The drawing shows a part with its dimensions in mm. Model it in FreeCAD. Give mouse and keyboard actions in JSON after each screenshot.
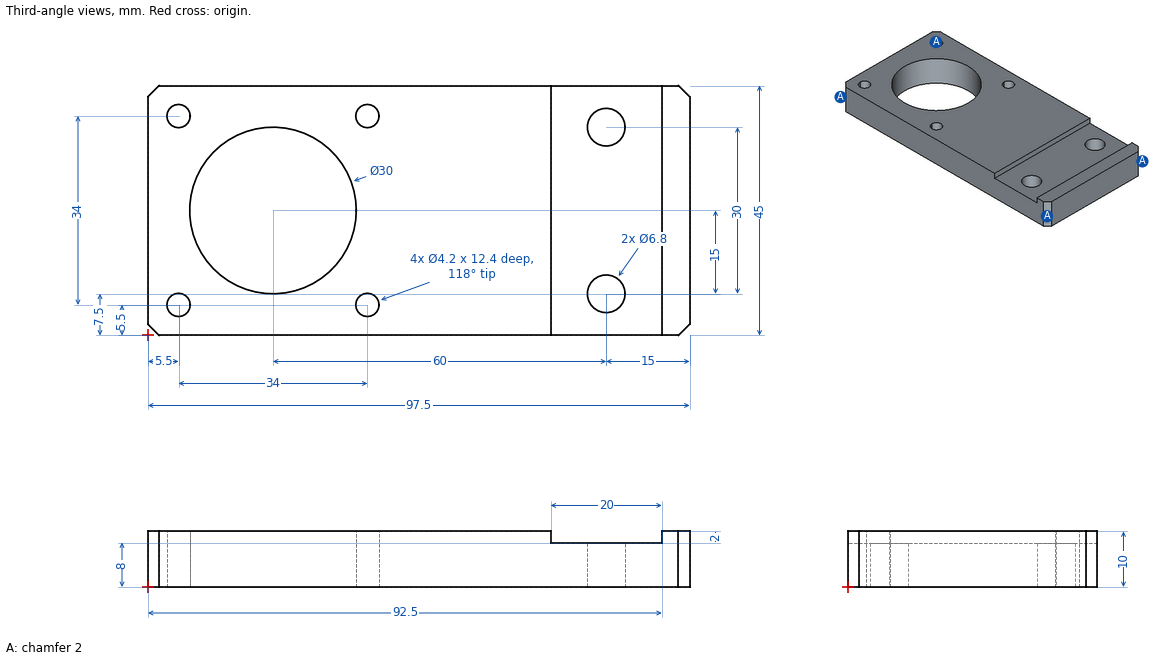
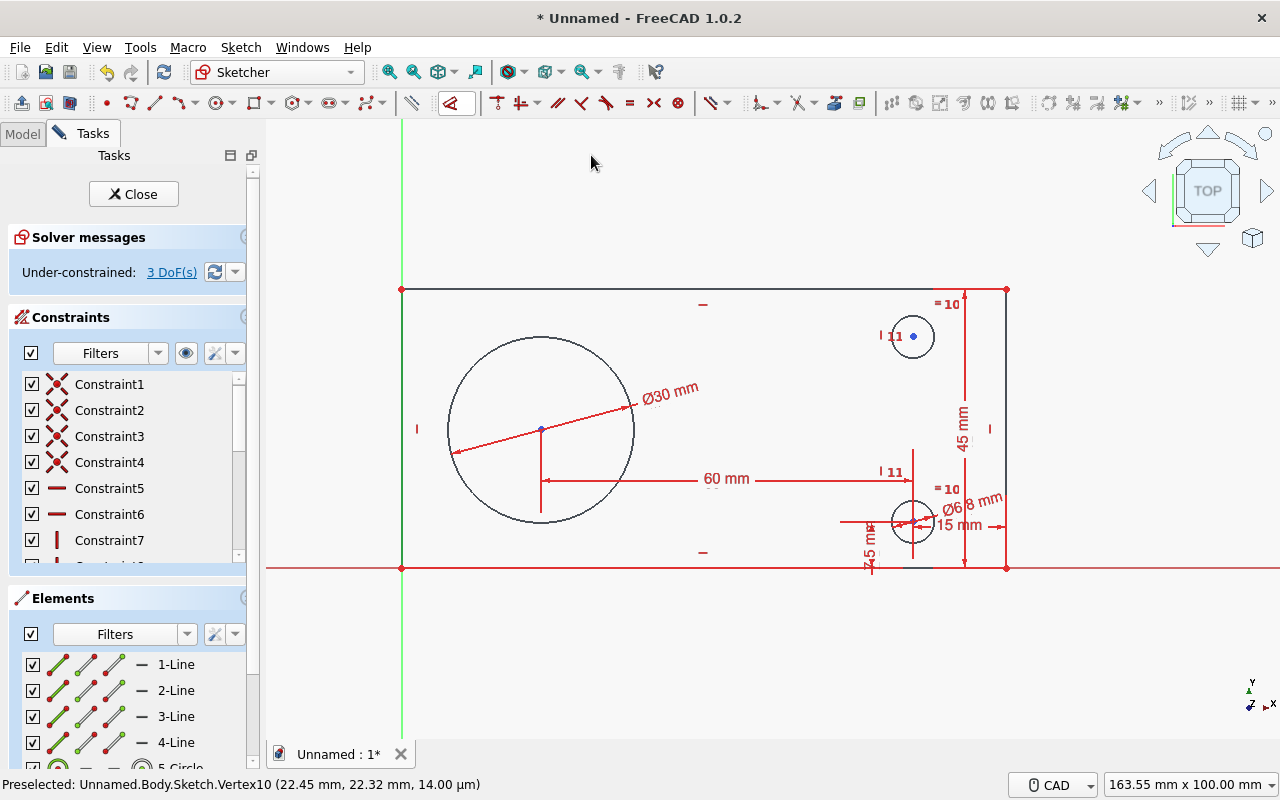
{"action": "left_click", "coordinate": [913, 522]}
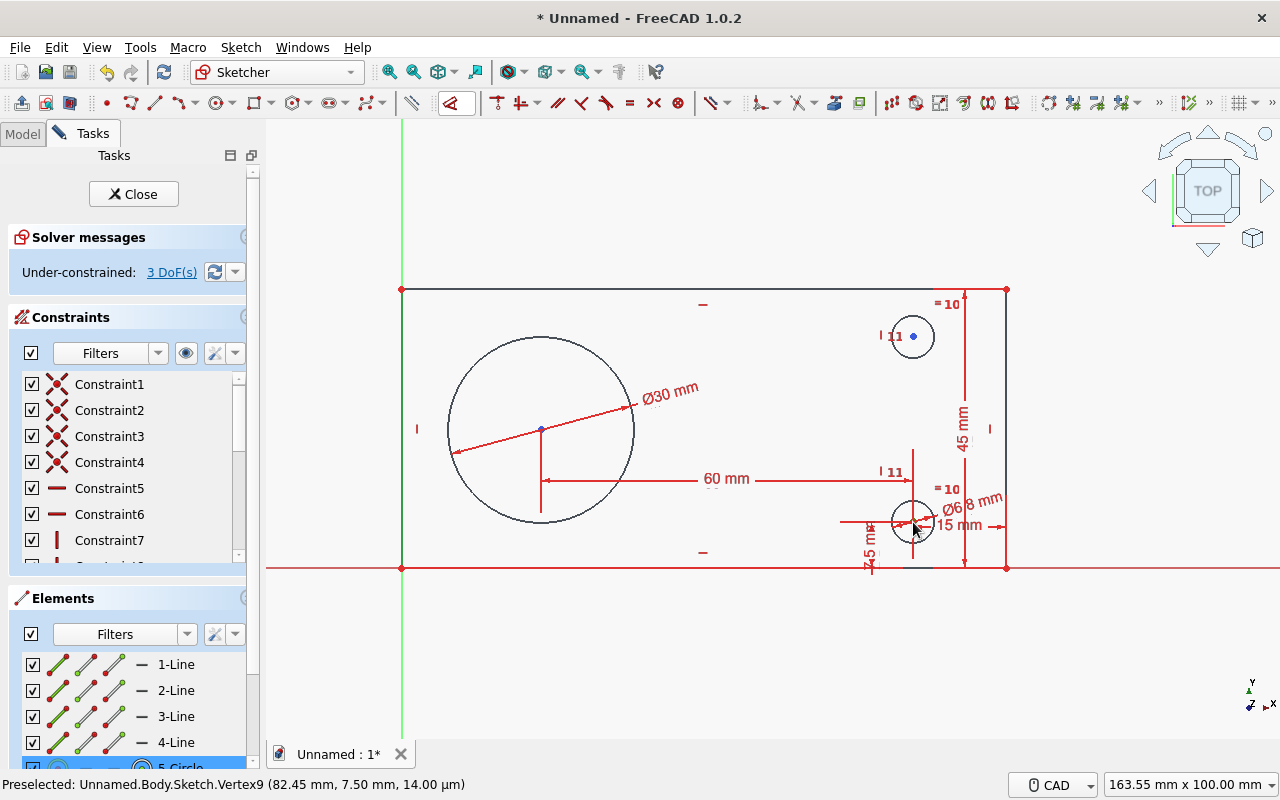
{"action": "left_click", "coordinate": [541, 430]}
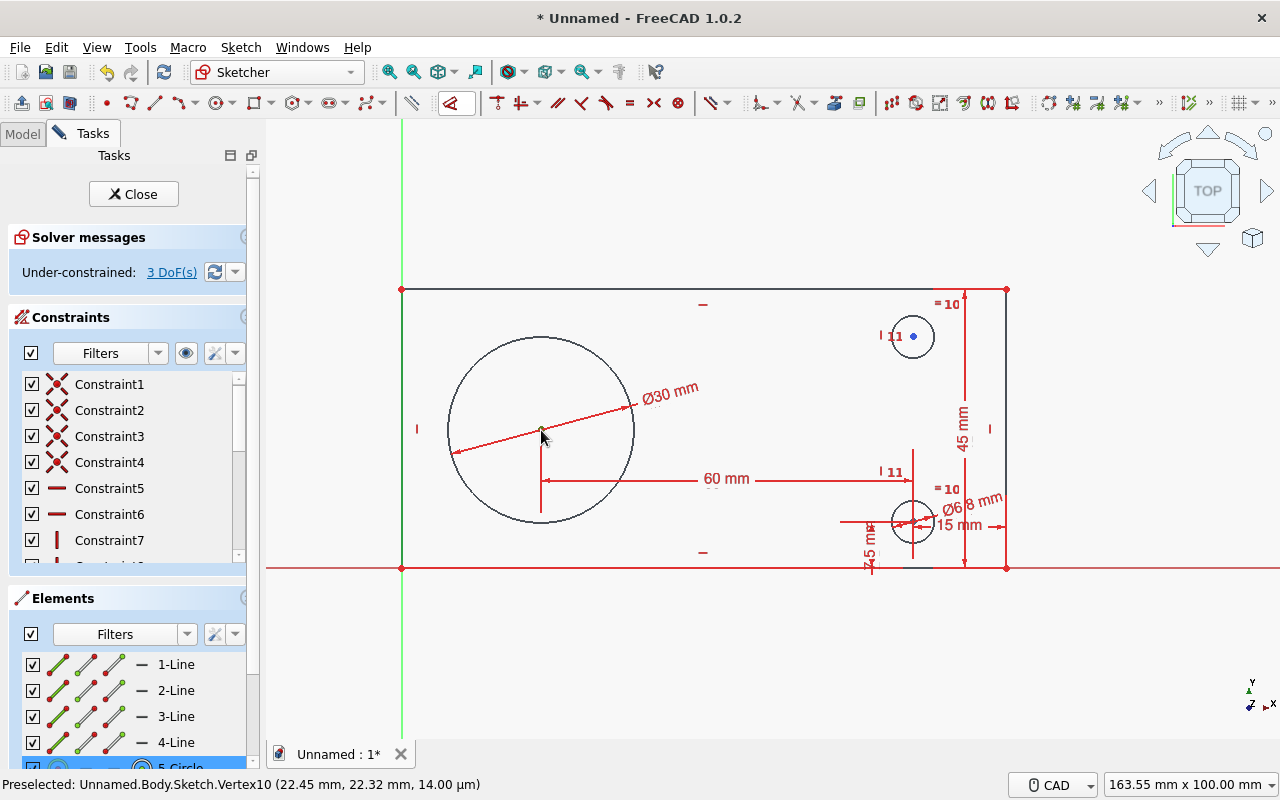
{"action": "left_click", "coordinate": [470, 104]}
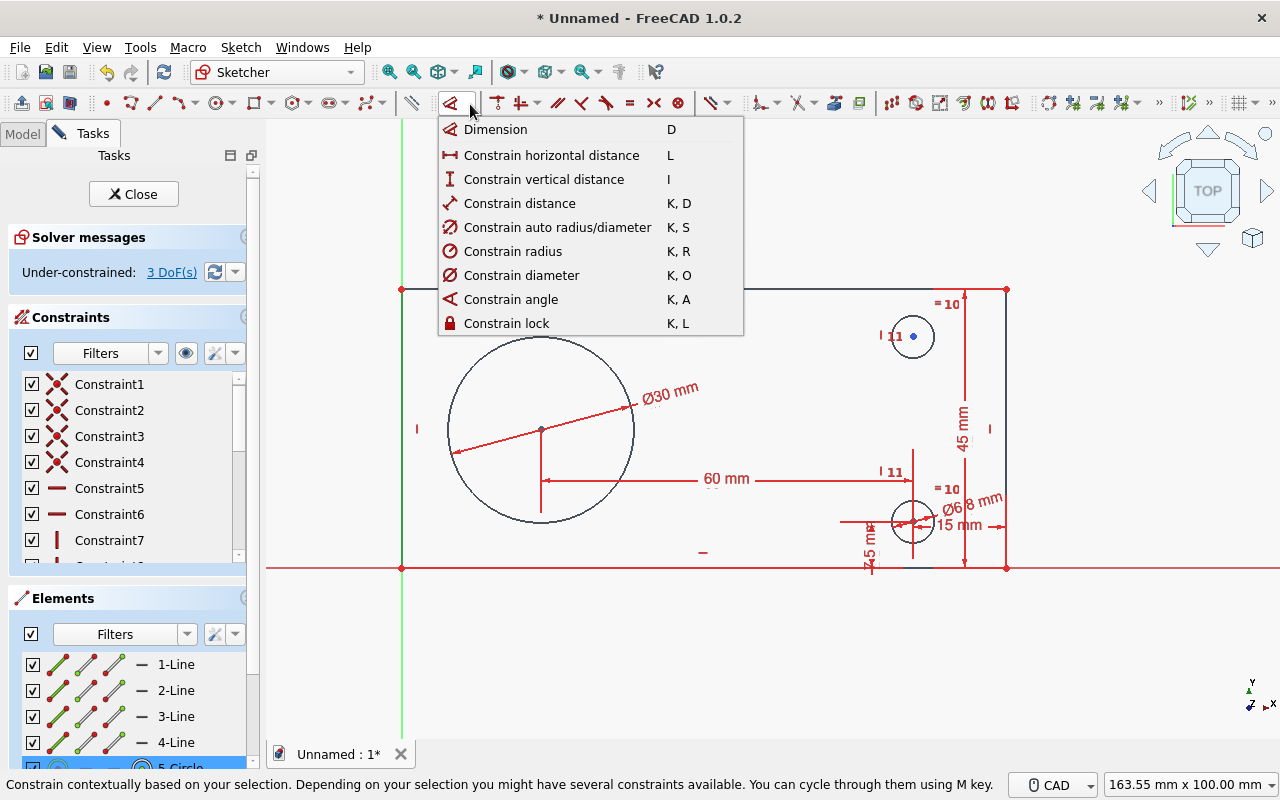
{"action": "left_click", "coordinate": [591, 179]}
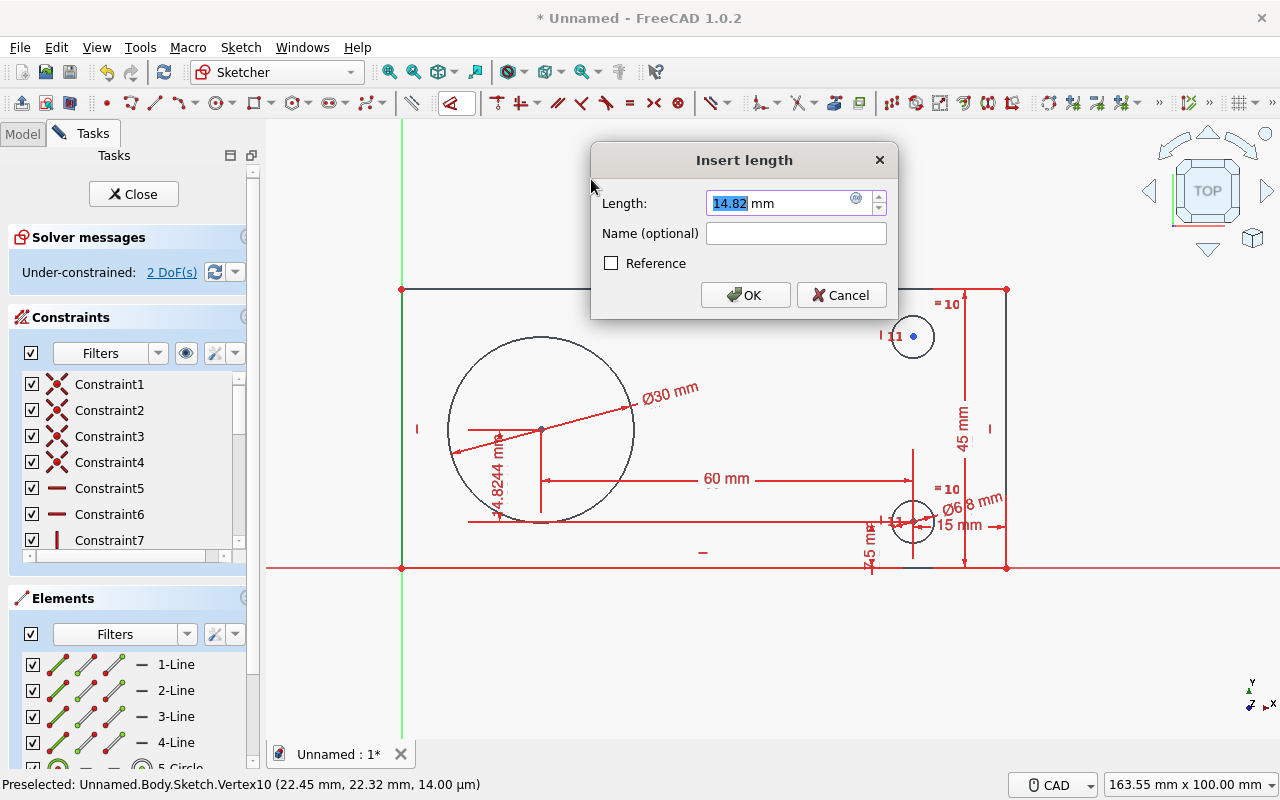
{"action": "type", "text": "15"}
{"action": "key", "text": "Return"}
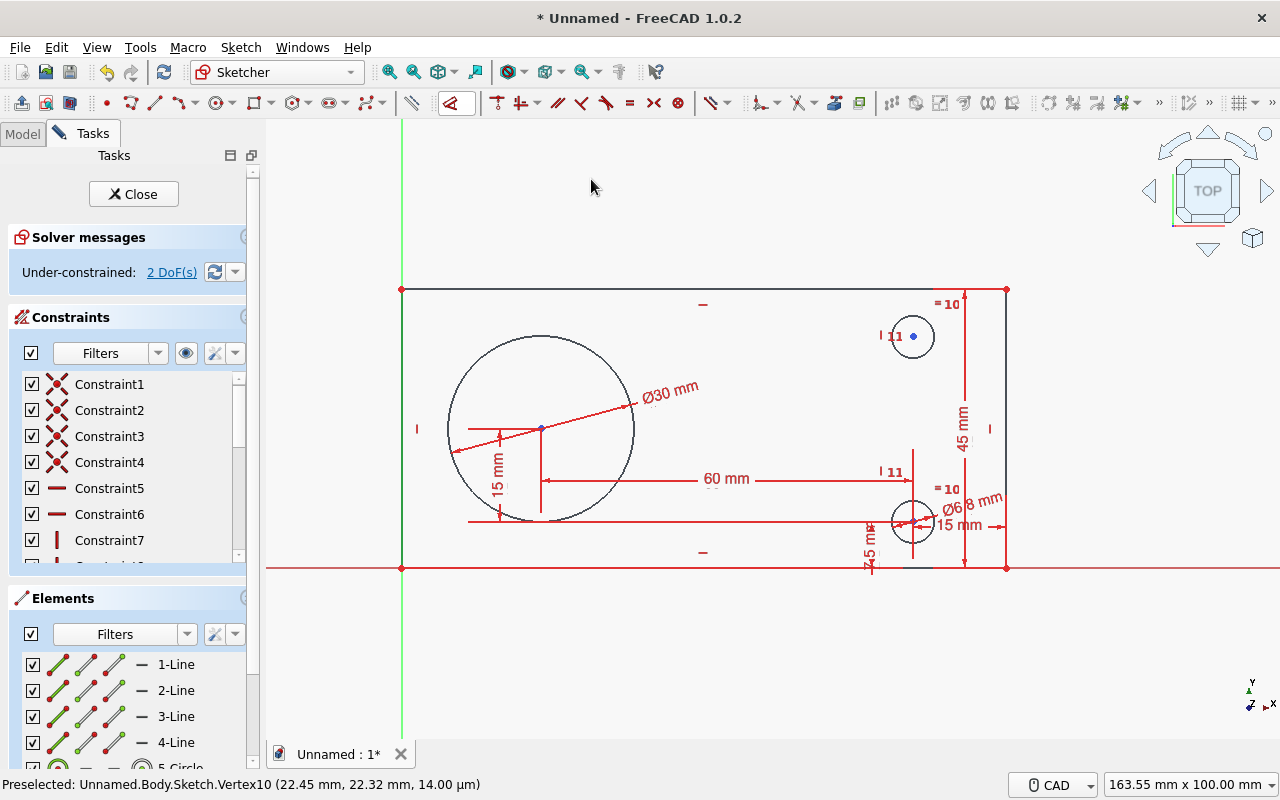
{"action": "left_click", "coordinate": [913, 522]}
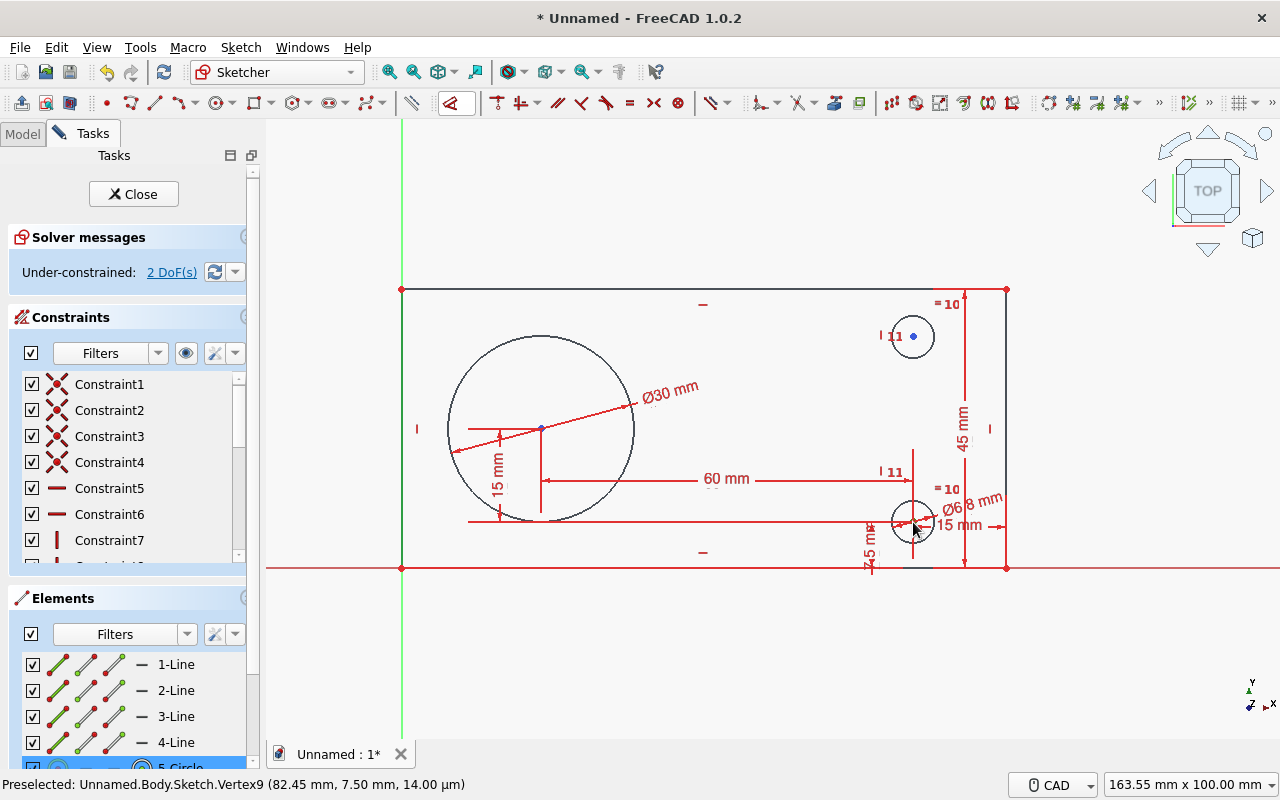
{"action": "left_click", "coordinate": [913, 337]}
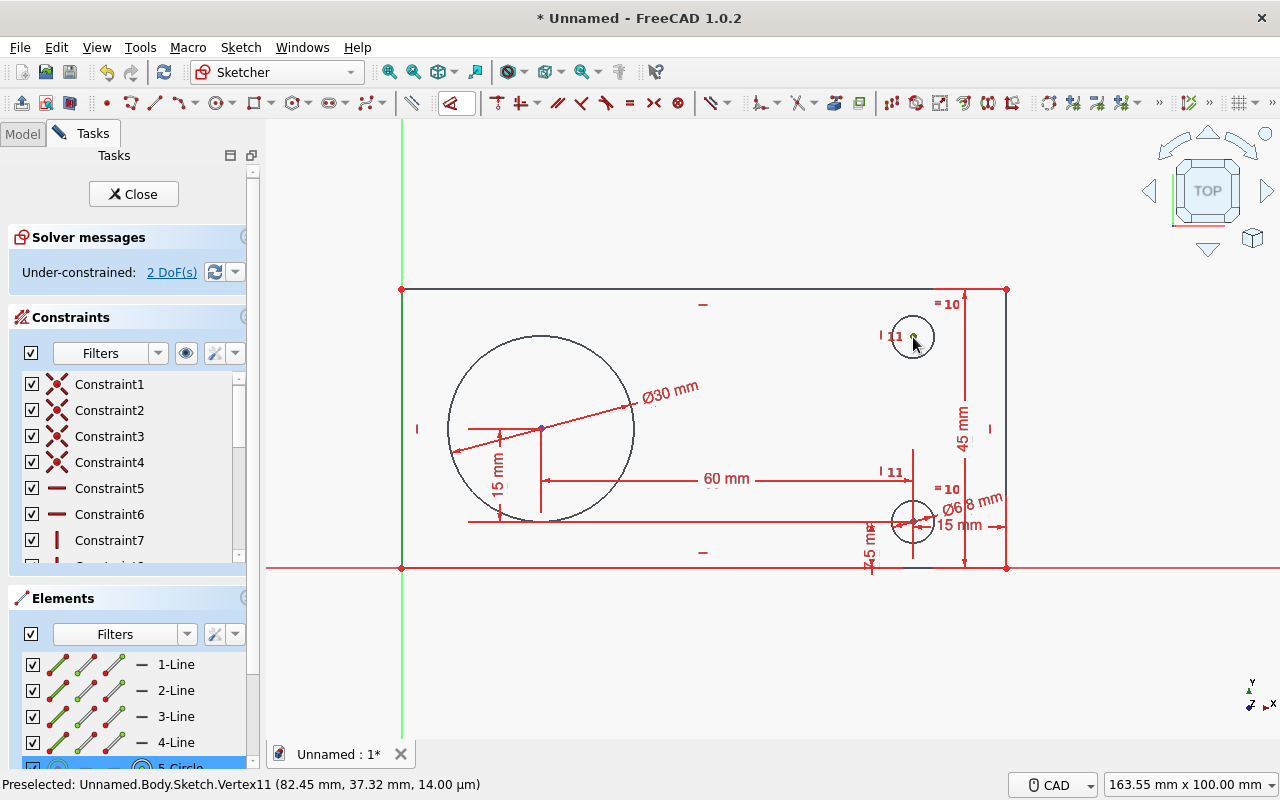
{"action": "key", "text": "i"}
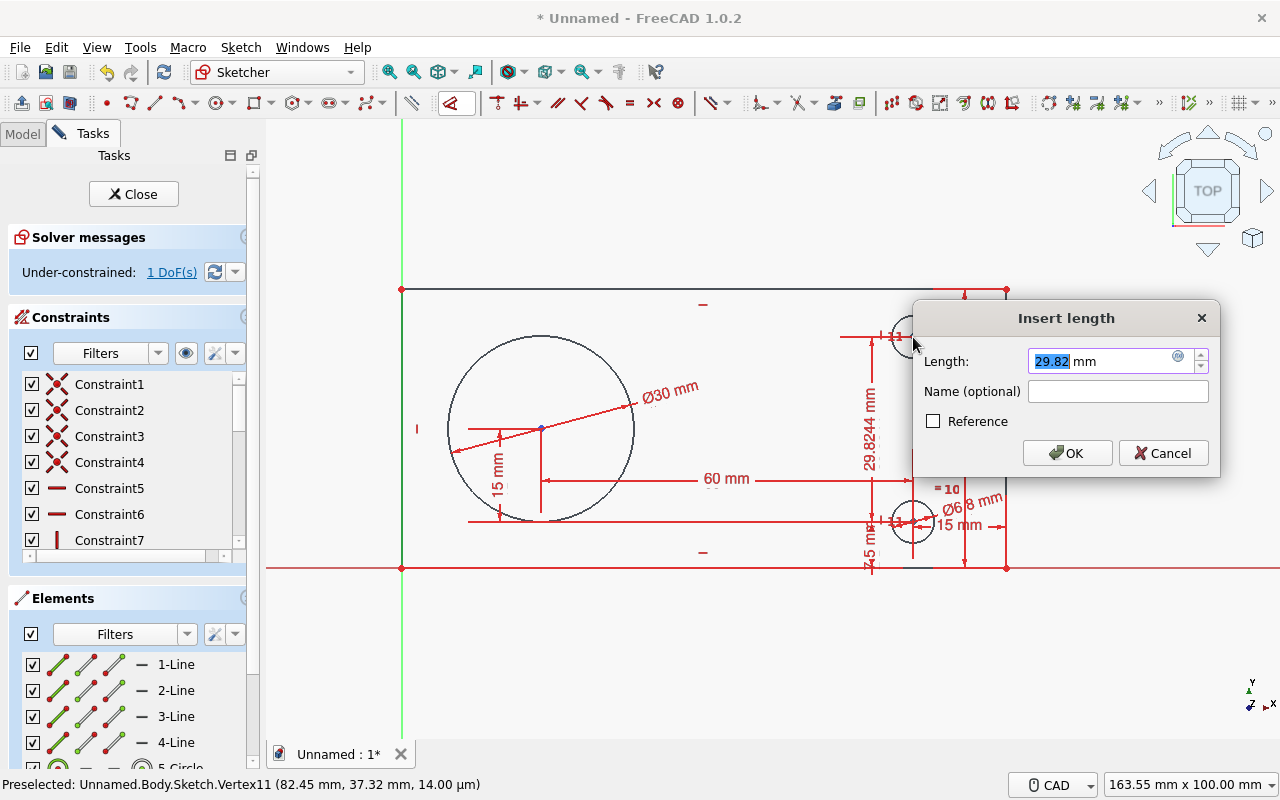
{"action": "type", "text": "30"}
{"action": "key", "text": "Return"}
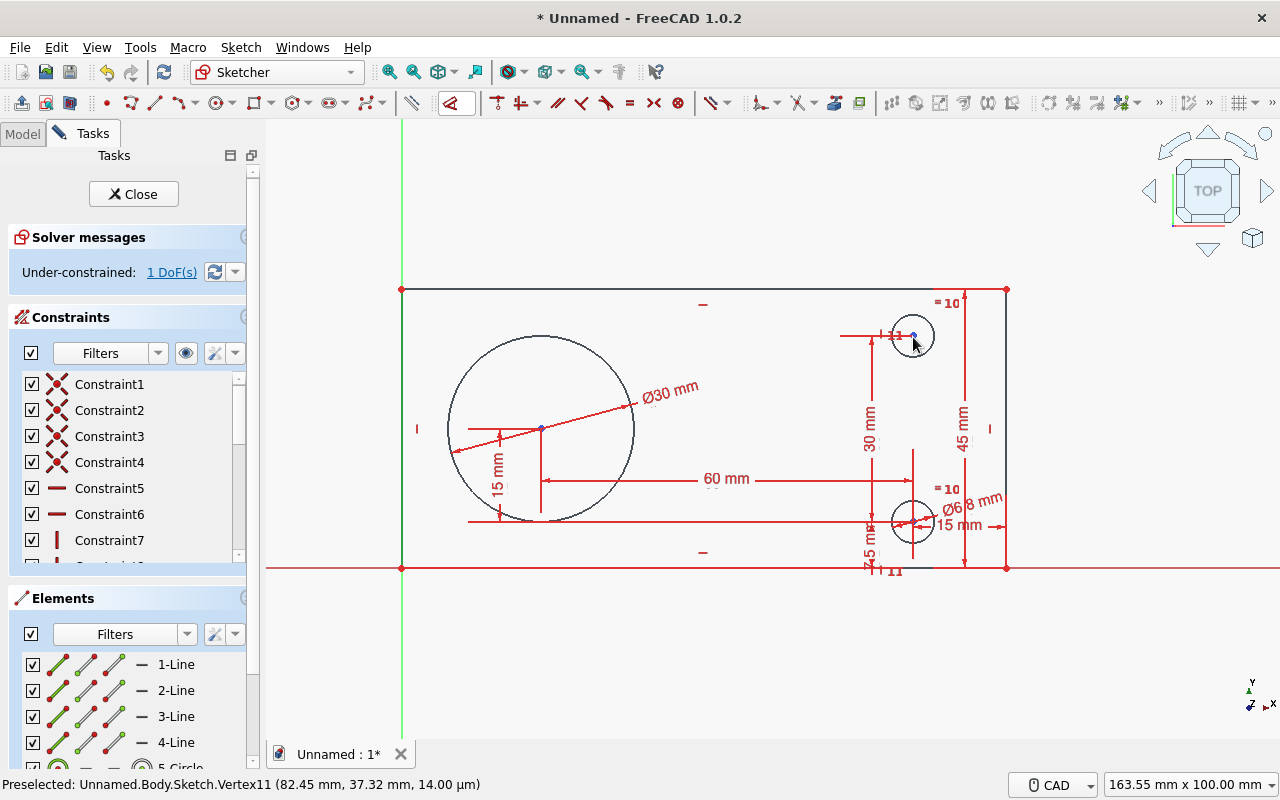
{"action": "left_click", "coordinate": [583, 568]}